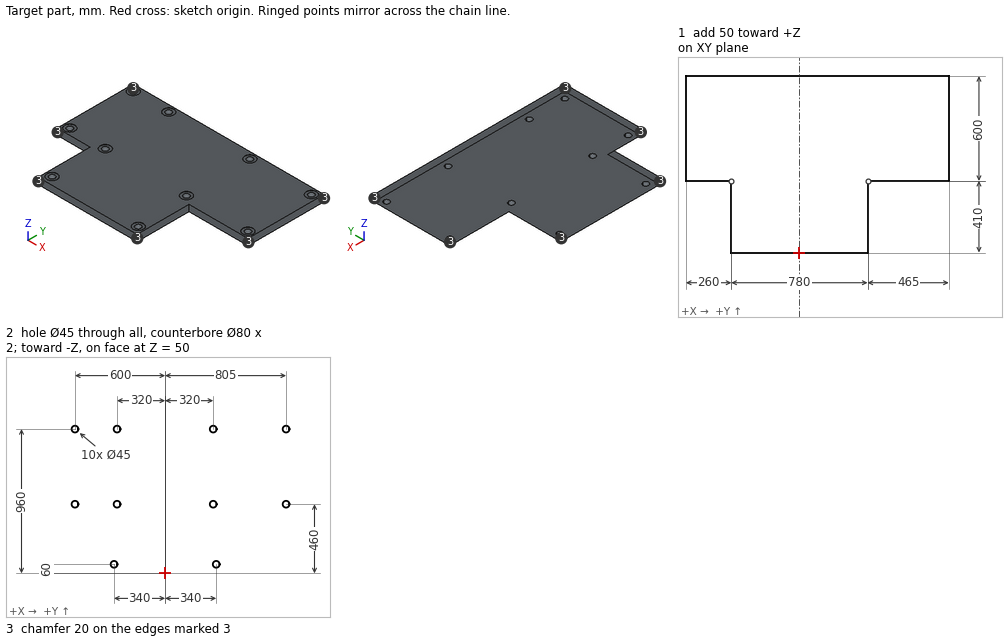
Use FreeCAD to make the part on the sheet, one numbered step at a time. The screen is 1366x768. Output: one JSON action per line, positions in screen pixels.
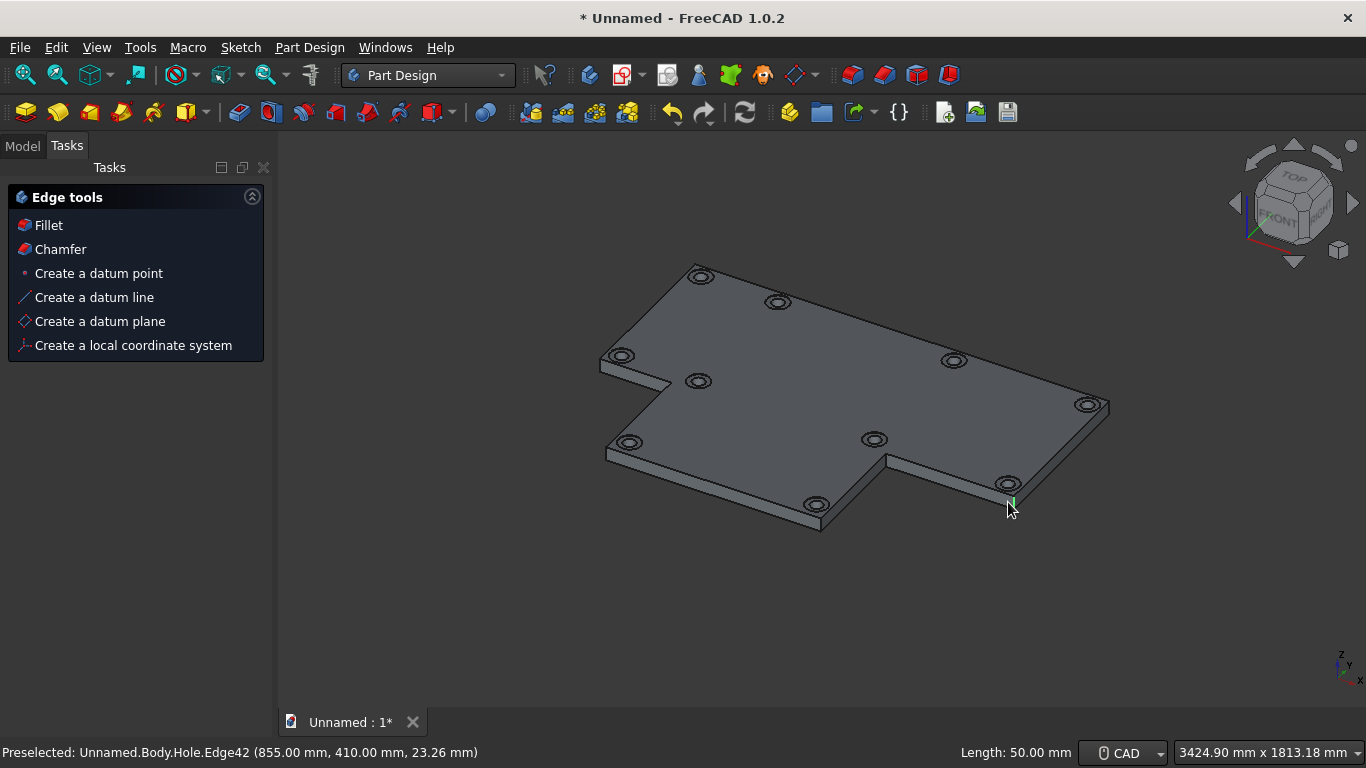
{"action": "left_click", "coordinate": [821, 524], "text": "ctrl"}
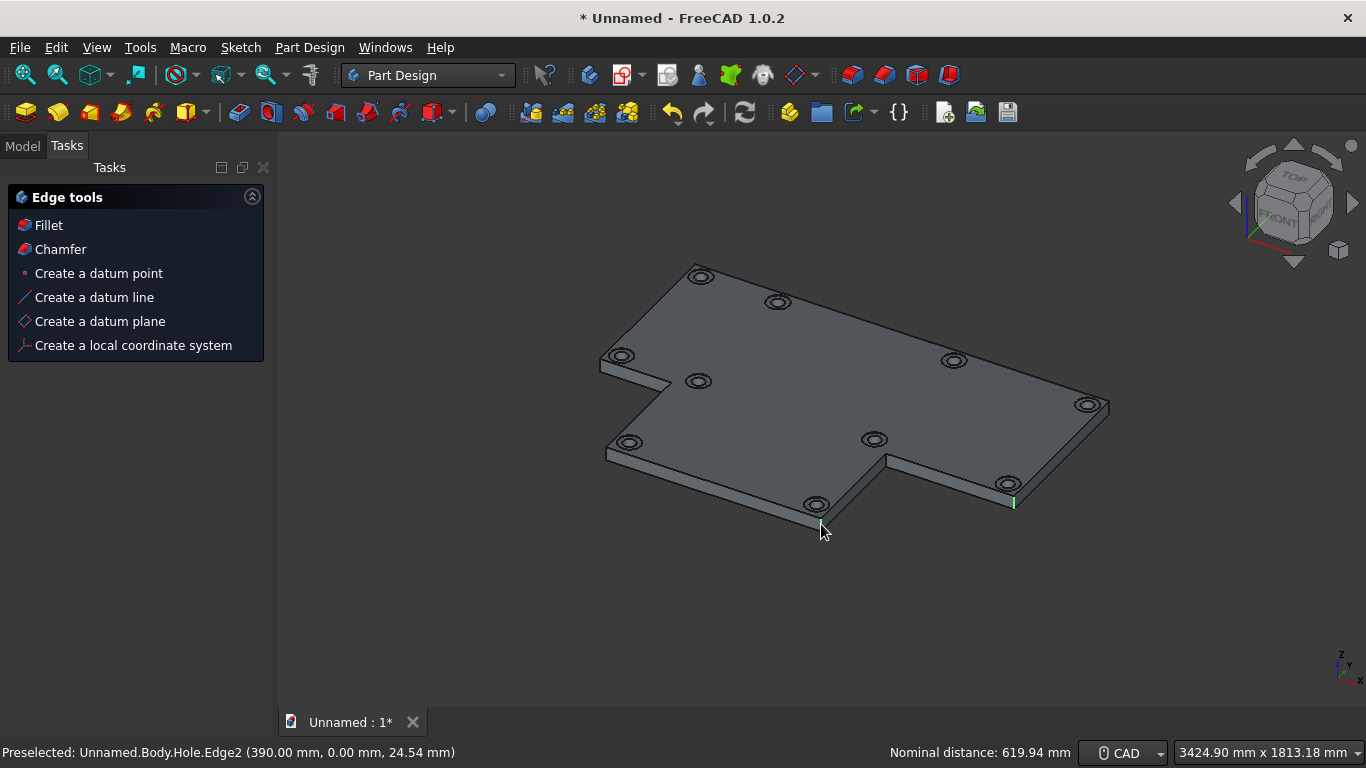
{"action": "scroll", "coordinate": [600, 364], "scroll_direction": "up", "scroll_amount": 5}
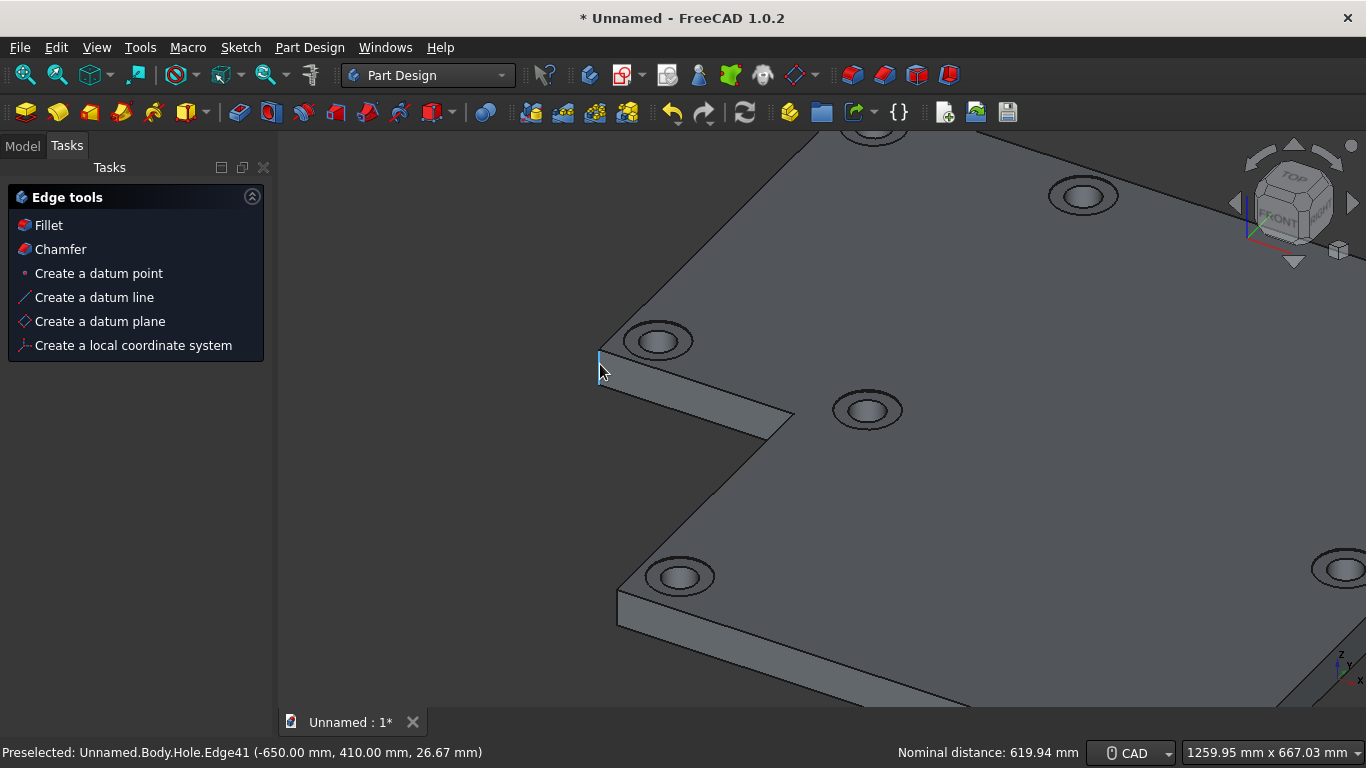
{"action": "left_click", "coordinate": [26, 76]}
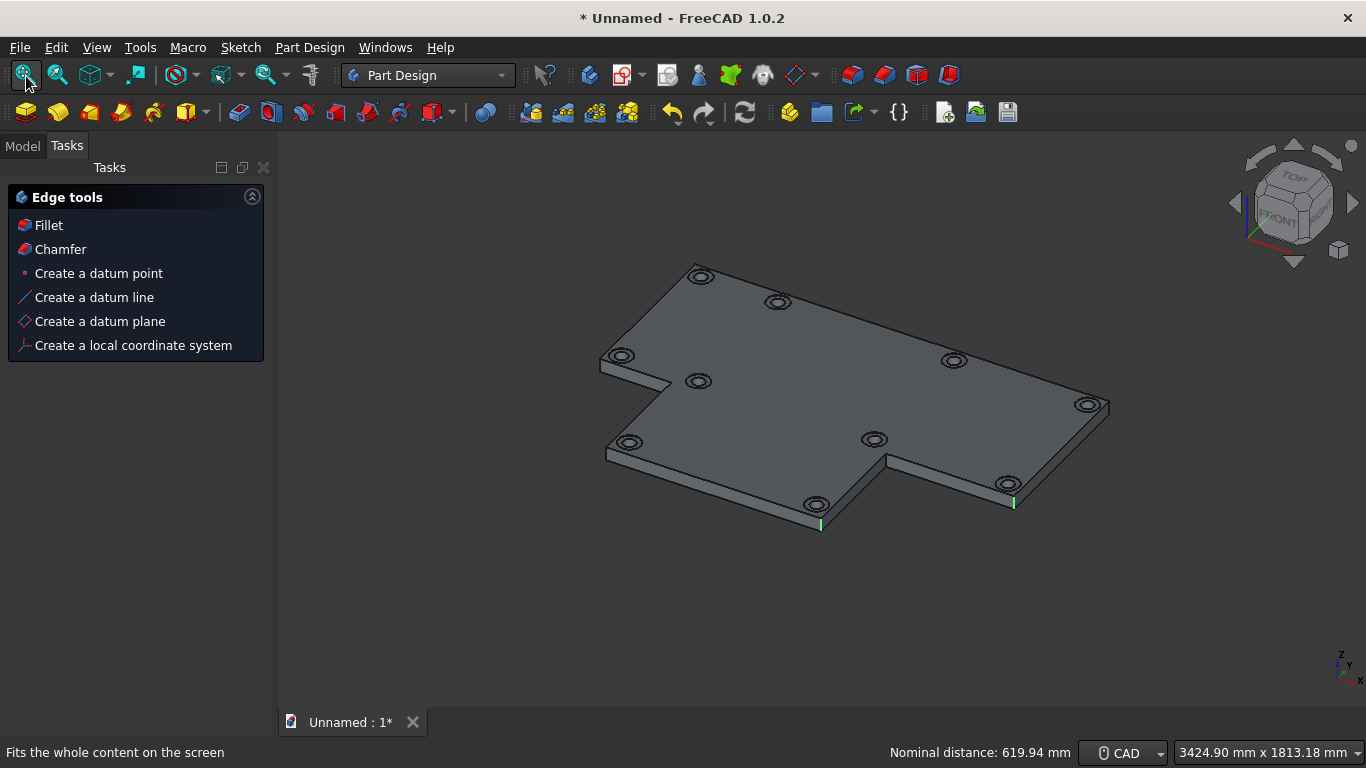
{"action": "key", "text": "0"}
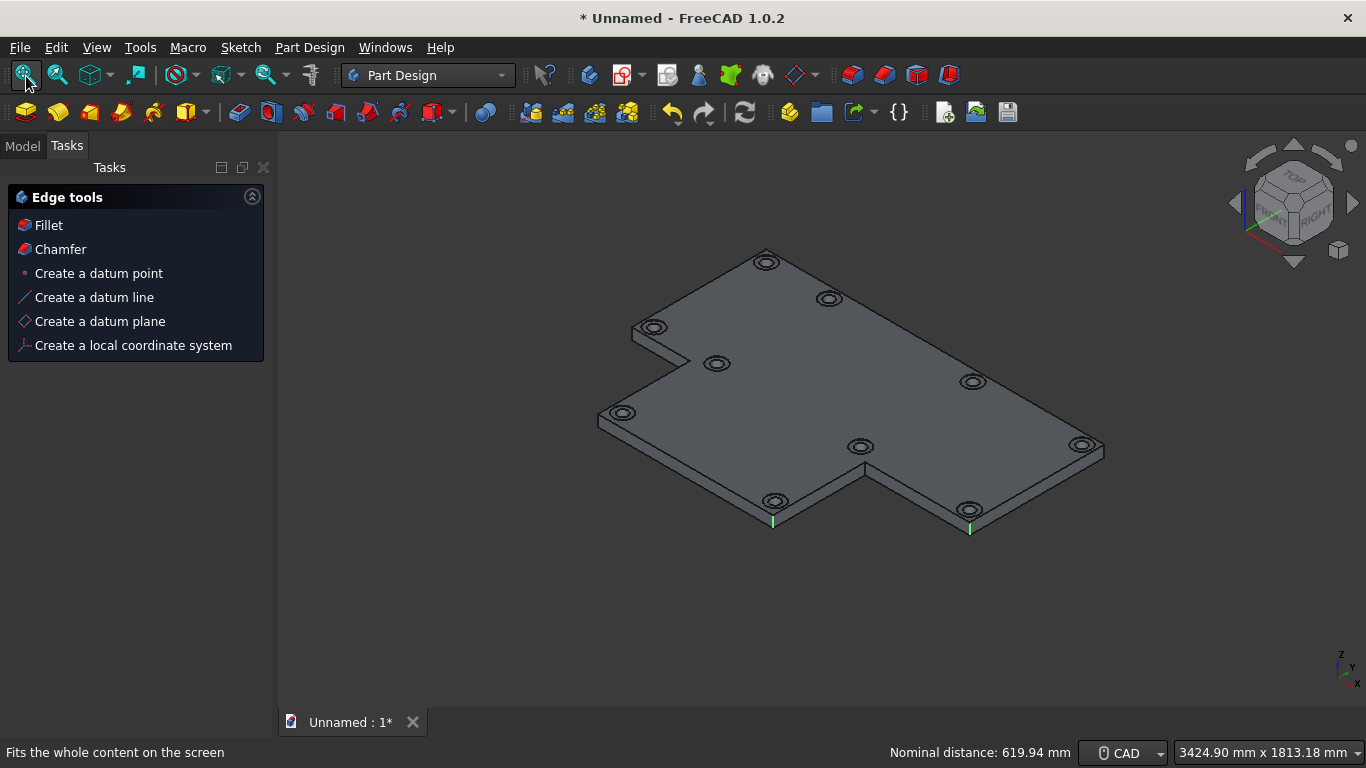
{"action": "scroll", "coordinate": [632, 333], "scroll_direction": "up", "scroll_amount": 5}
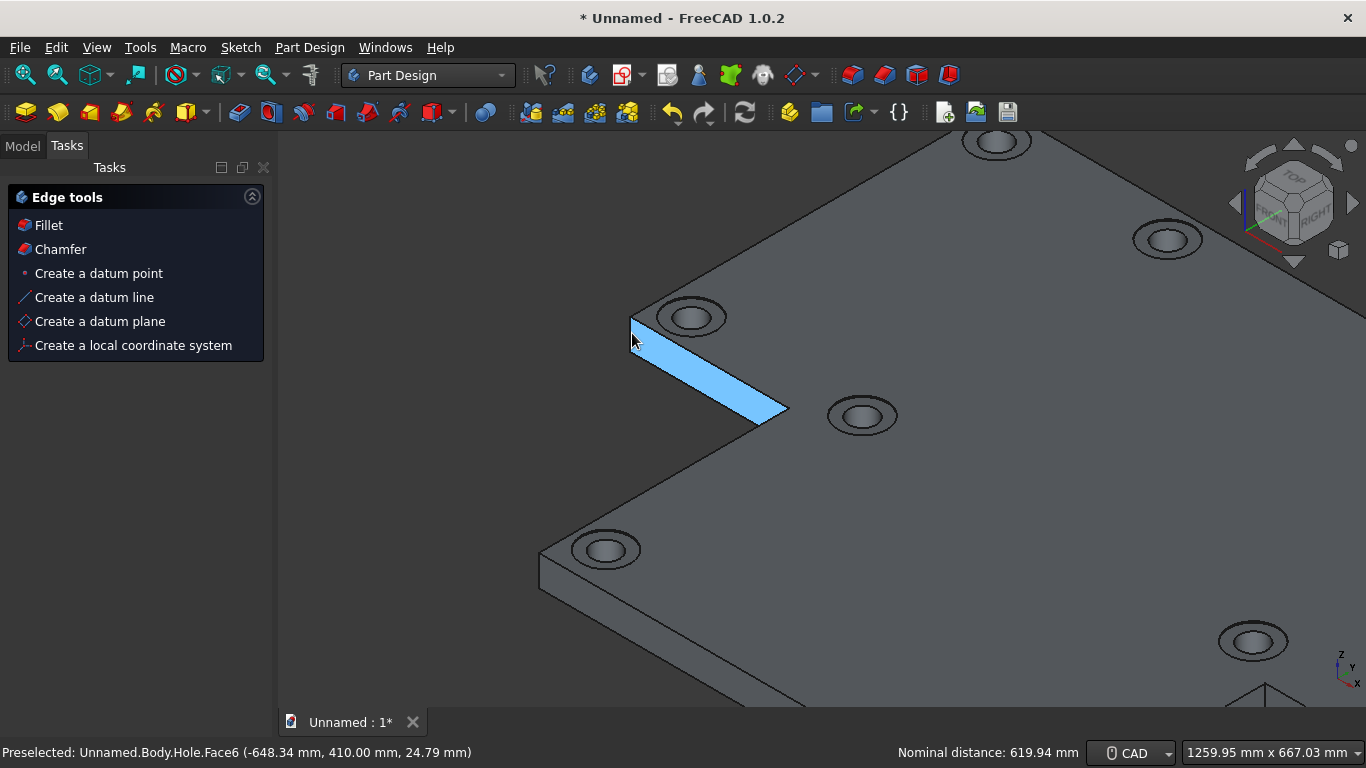
{"action": "key", "text": "v f"}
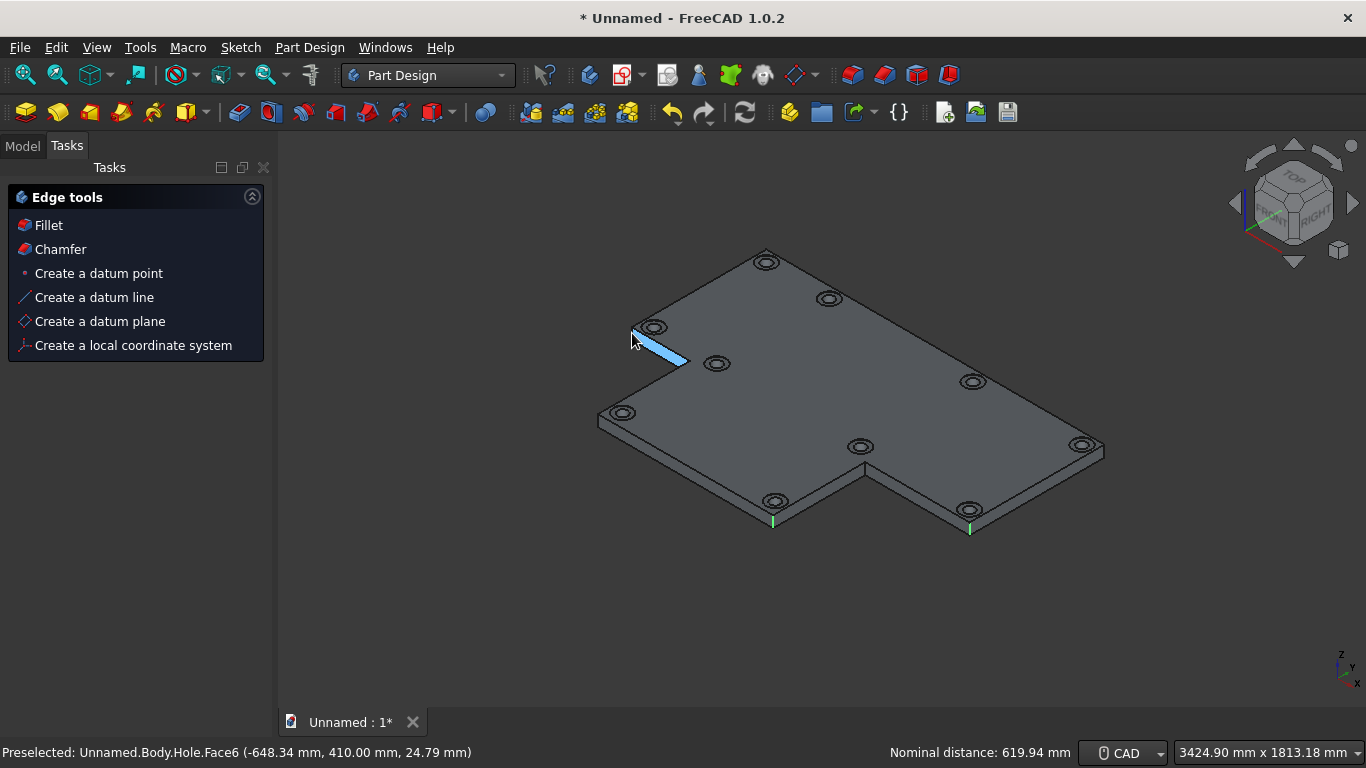
{"action": "key", "text": "2"}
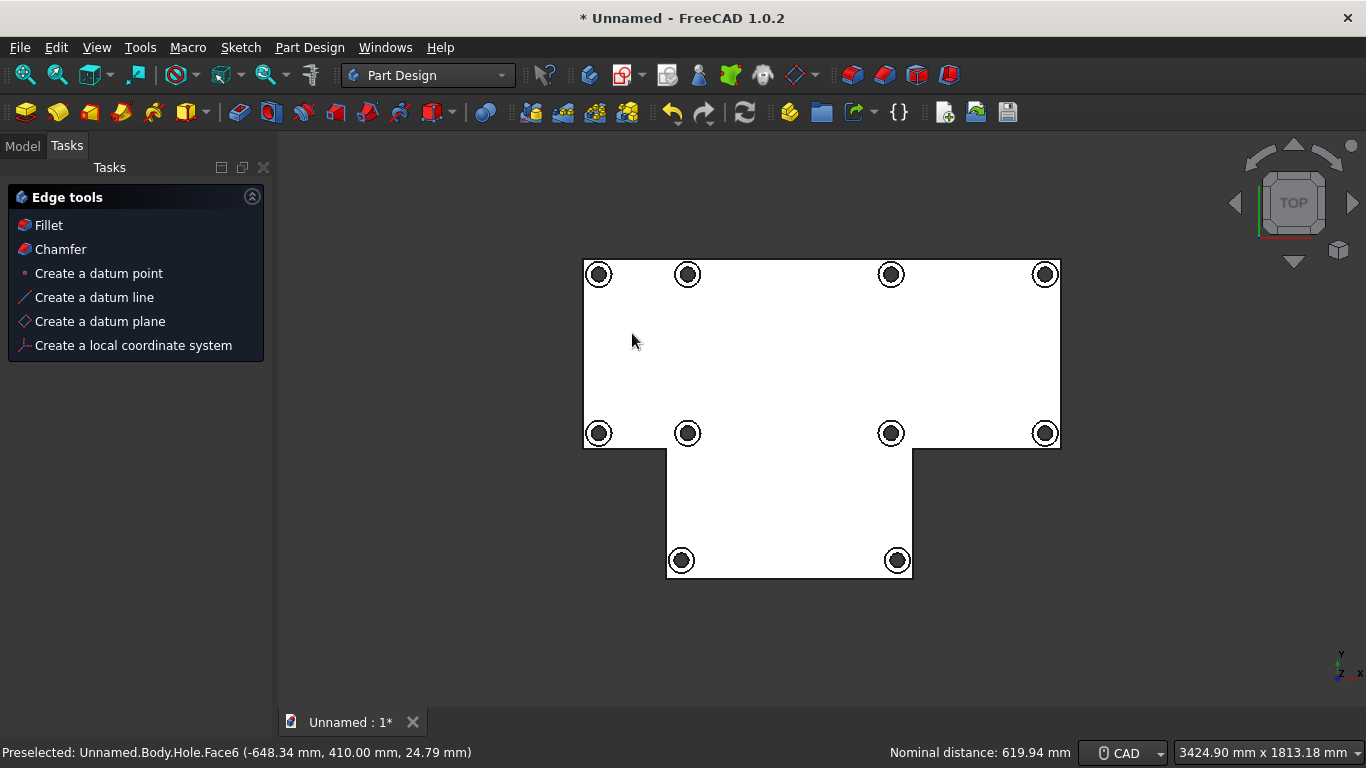
{"action": "scroll", "coordinate": [583, 448], "scroll_direction": "up", "scroll_amount": 5}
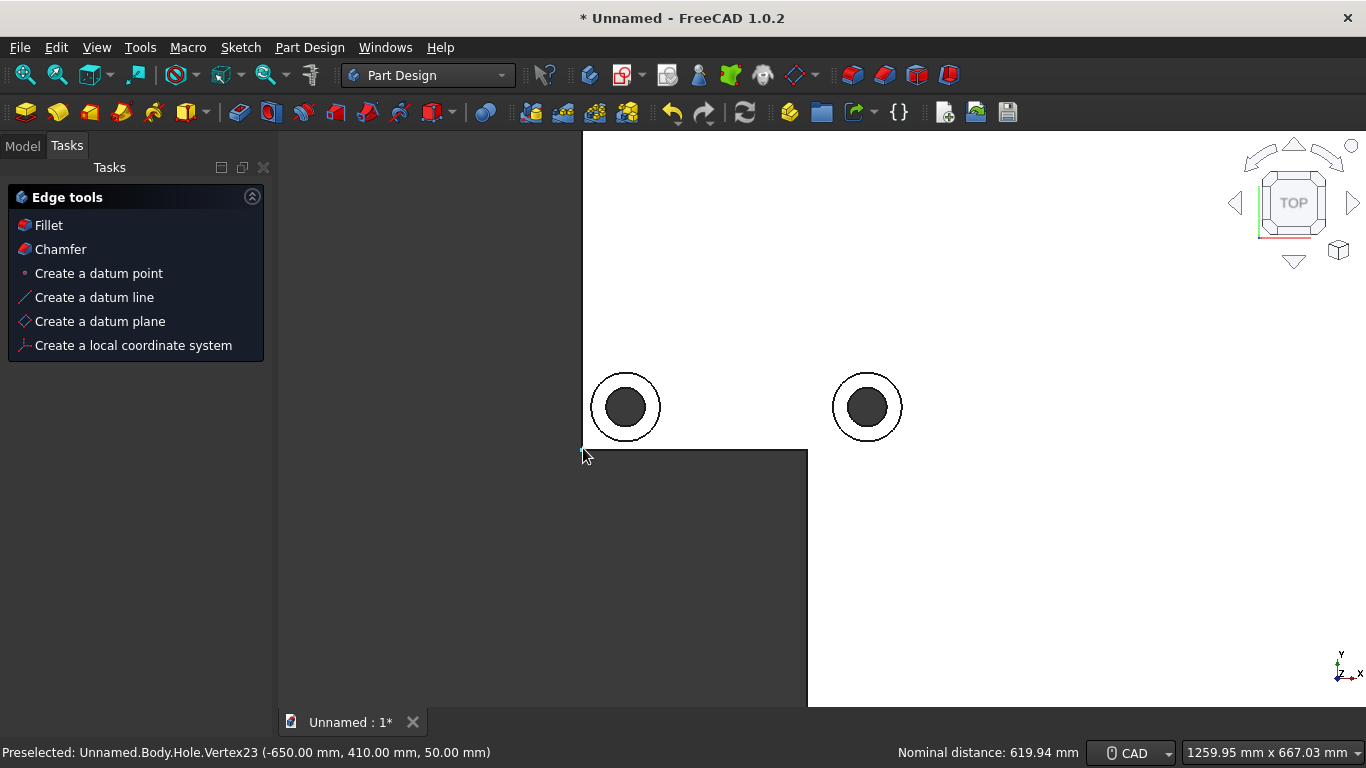
{"action": "left_click", "coordinate": [26, 76]}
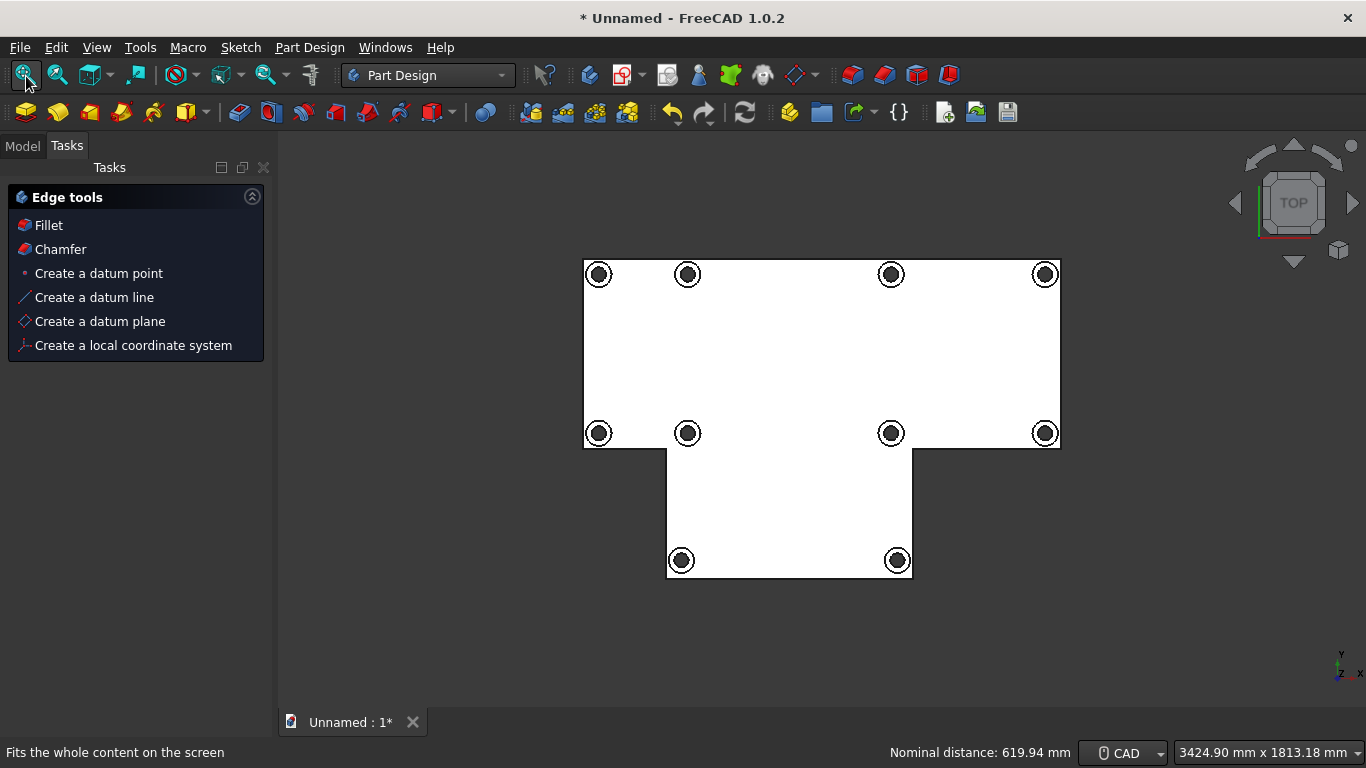
{"action": "key", "text": "1"}